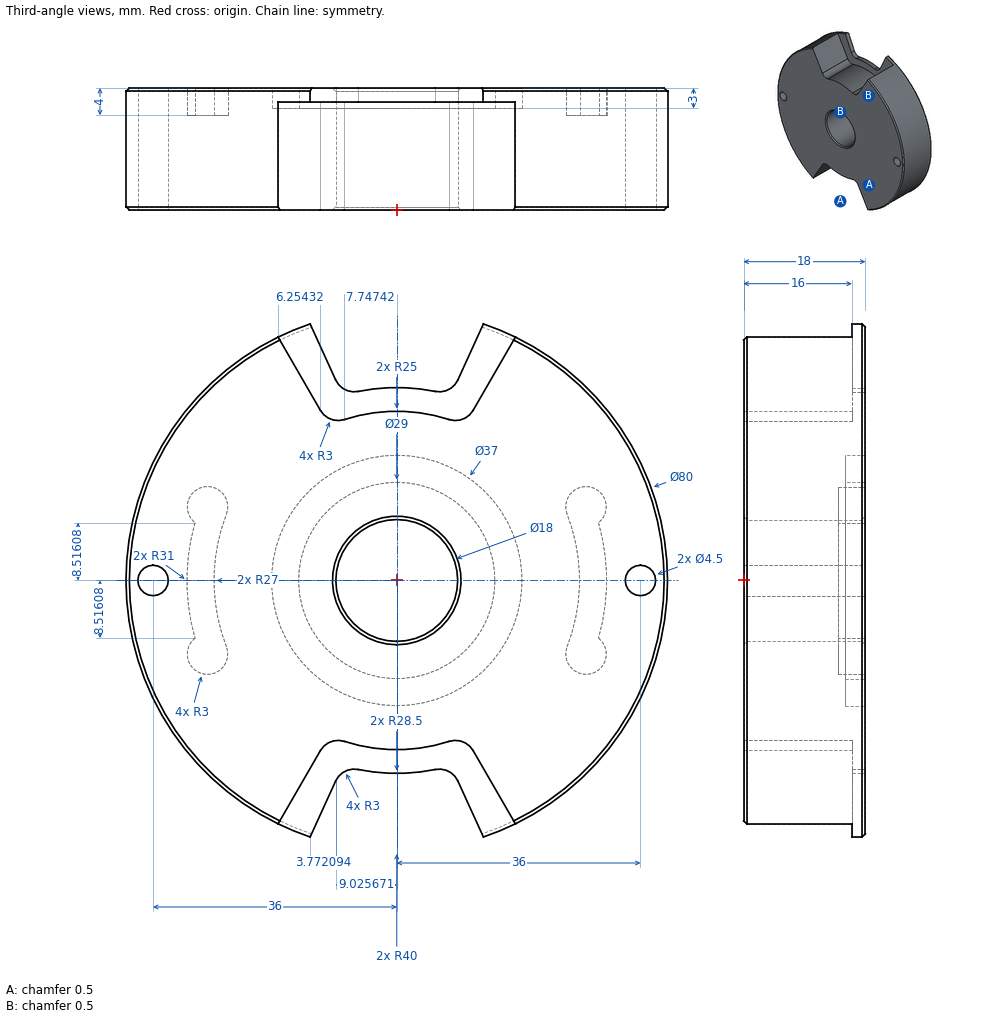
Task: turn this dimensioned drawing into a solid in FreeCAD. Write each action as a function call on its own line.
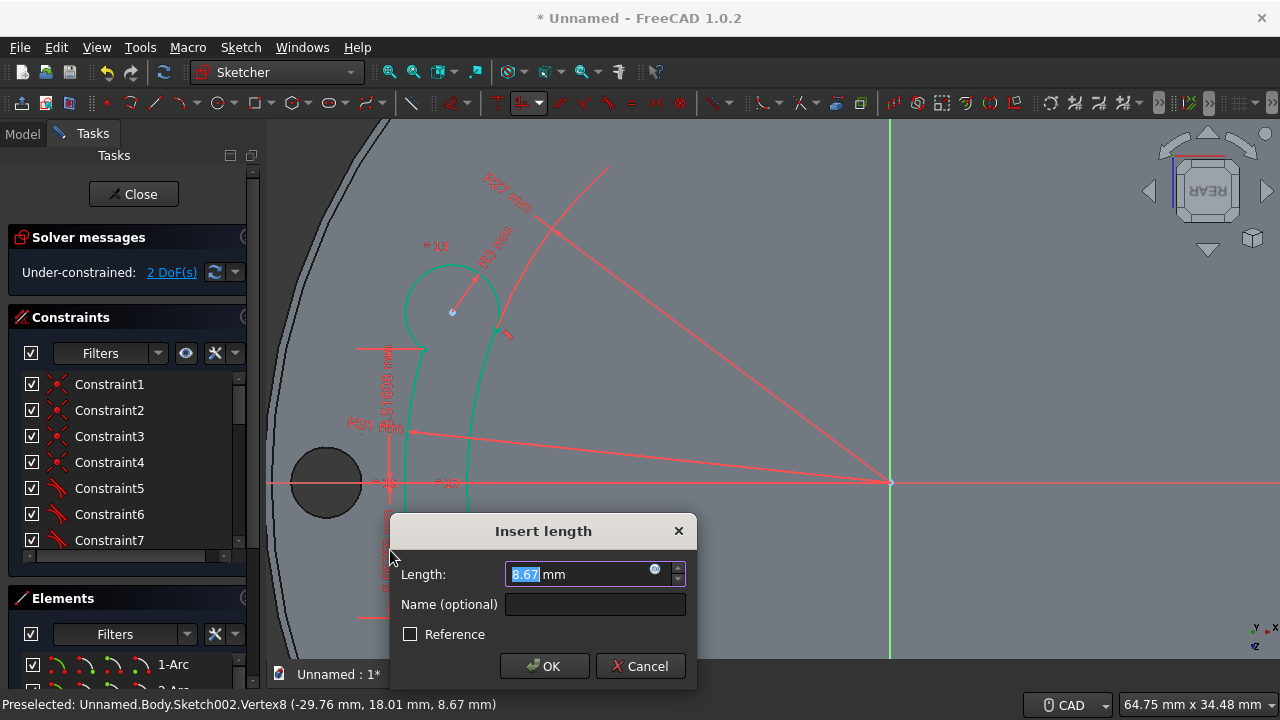
text(8.51608)
key(Return)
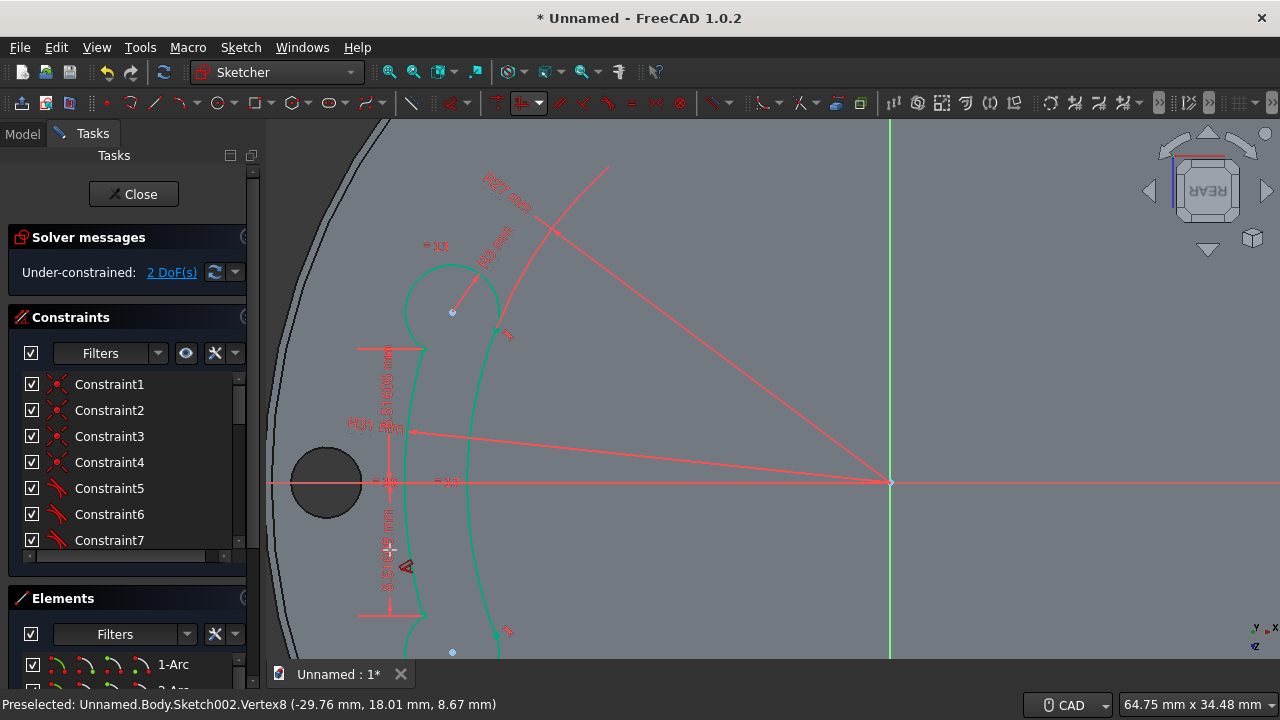
scroll(479, 275, down, 3)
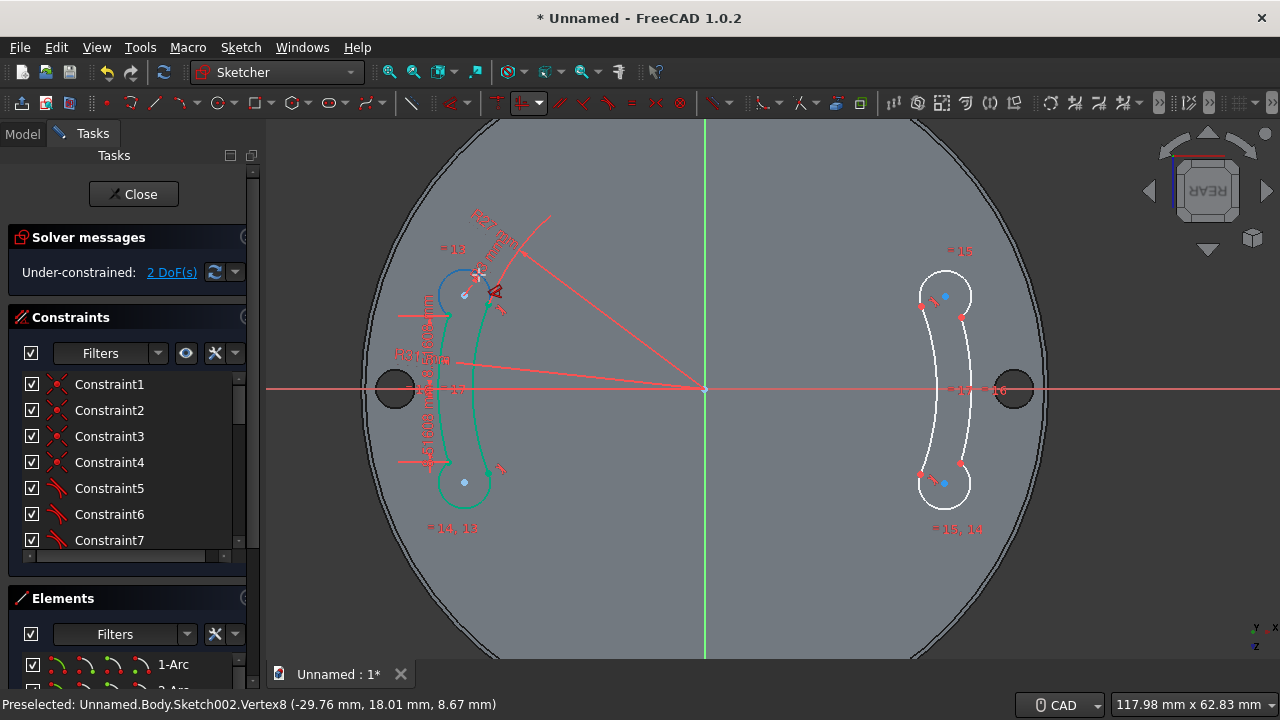
click(961, 463)
click(995, 426)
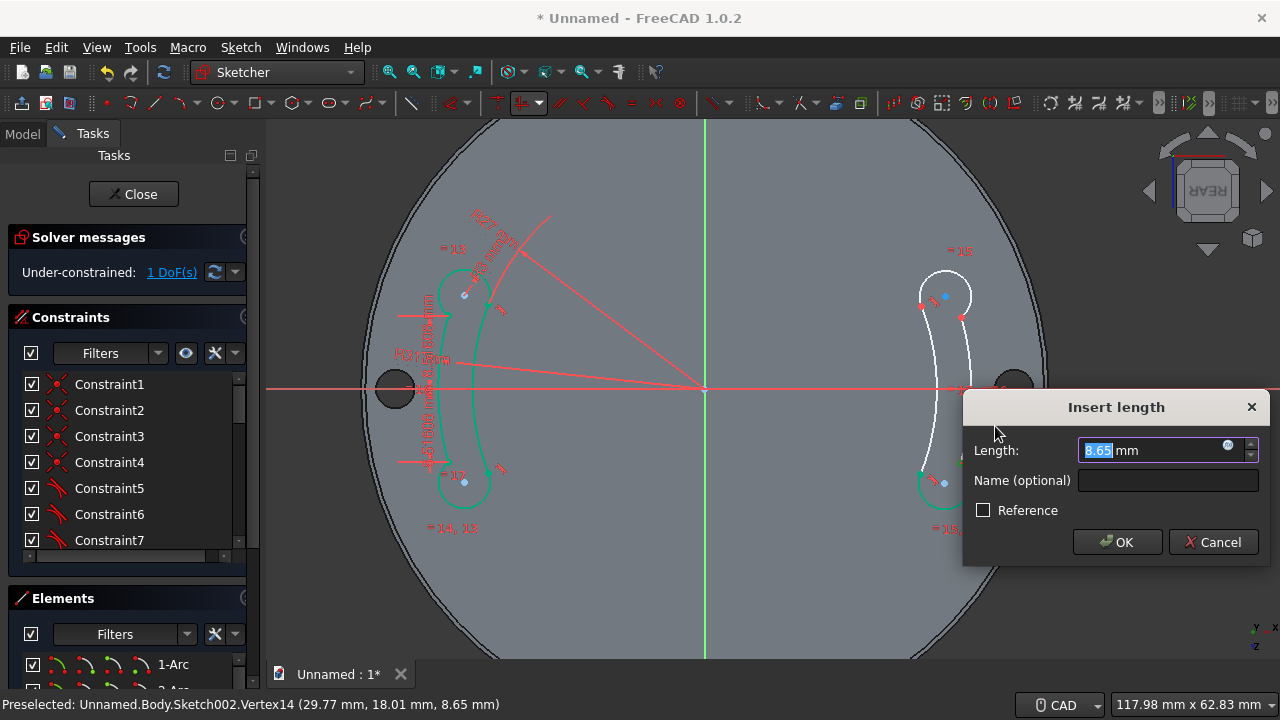
text(8.51608)
key(Return)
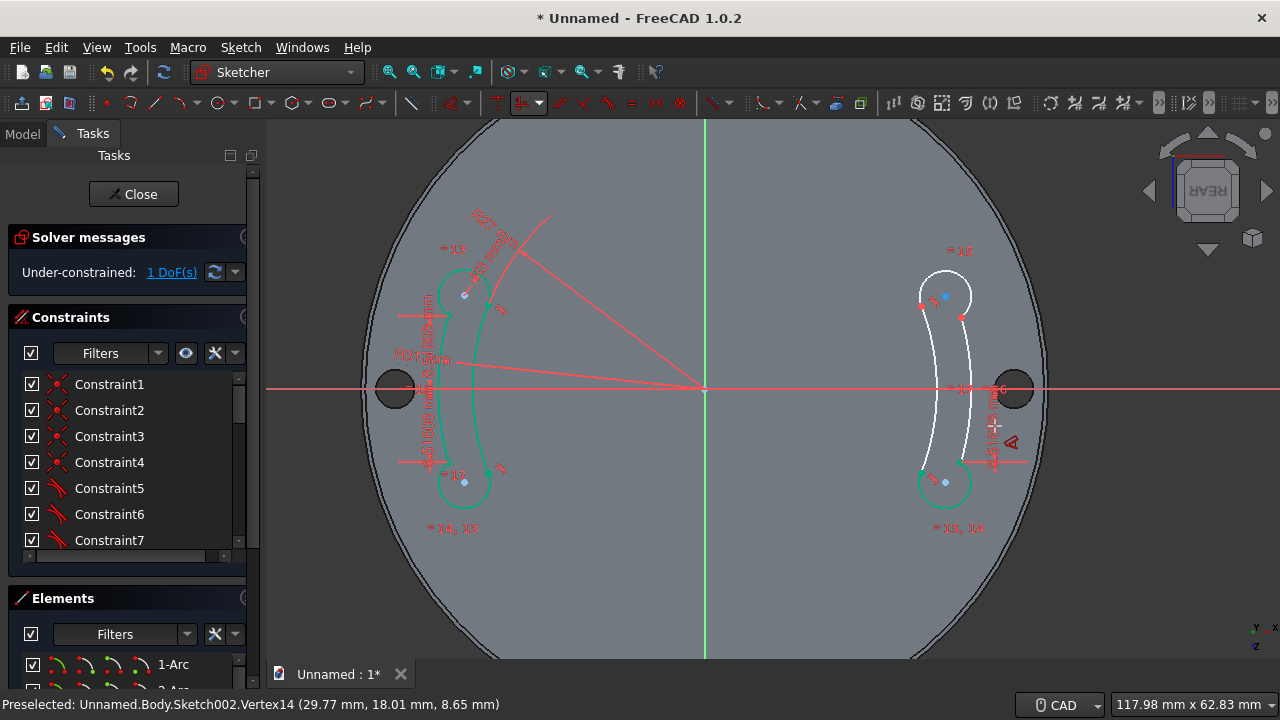
click(961, 317)
click(995, 353)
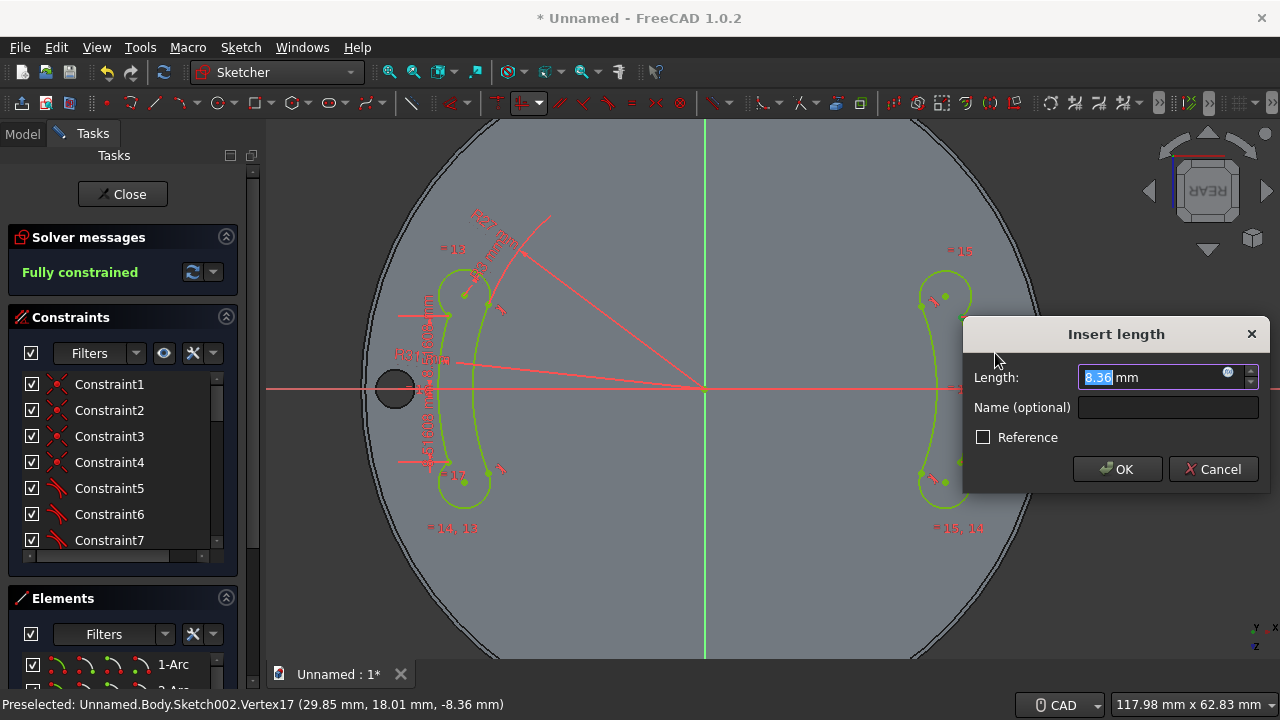
text(8.51608)
key(Return)
key(Escape)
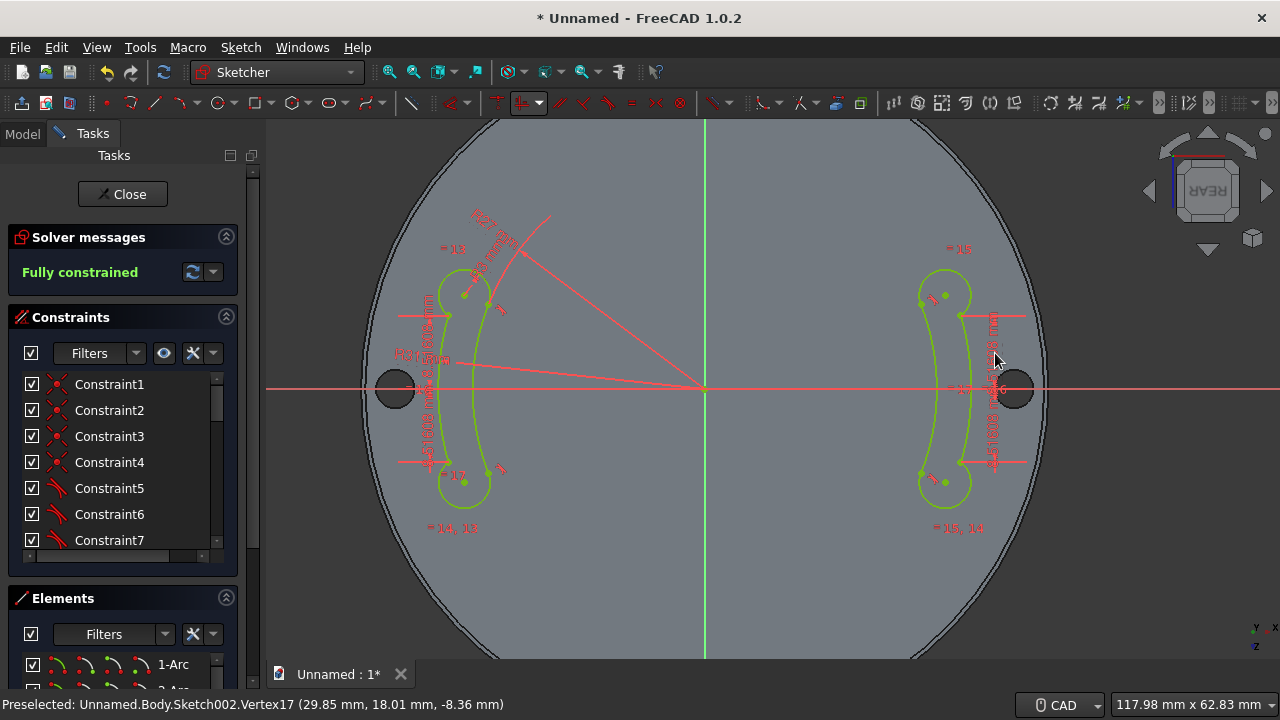
click(123, 194)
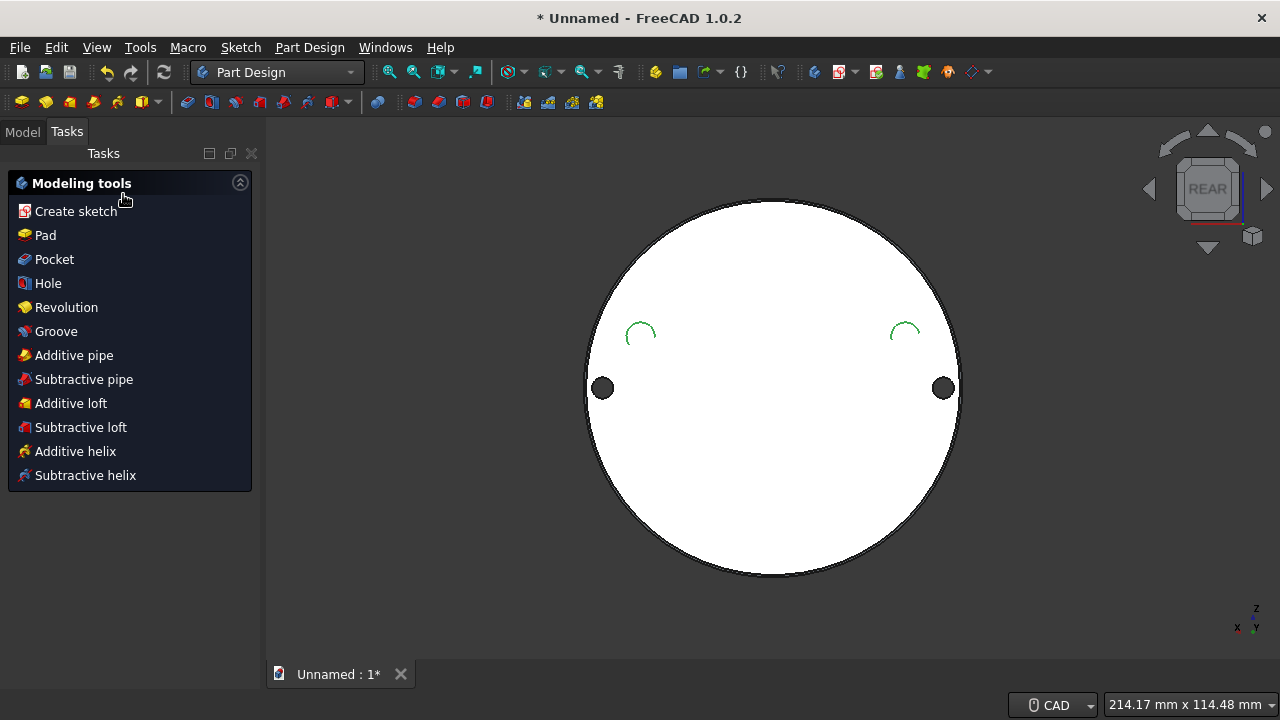
click(188, 102)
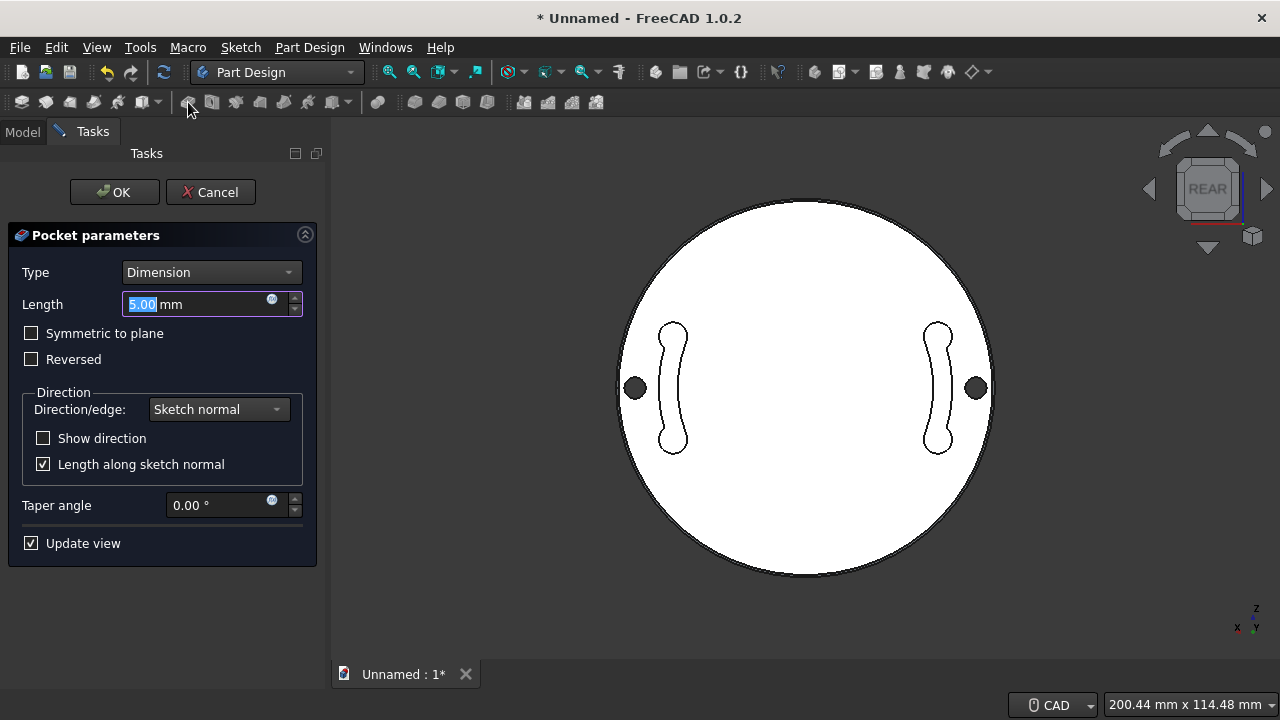
text(4)
key(Tab)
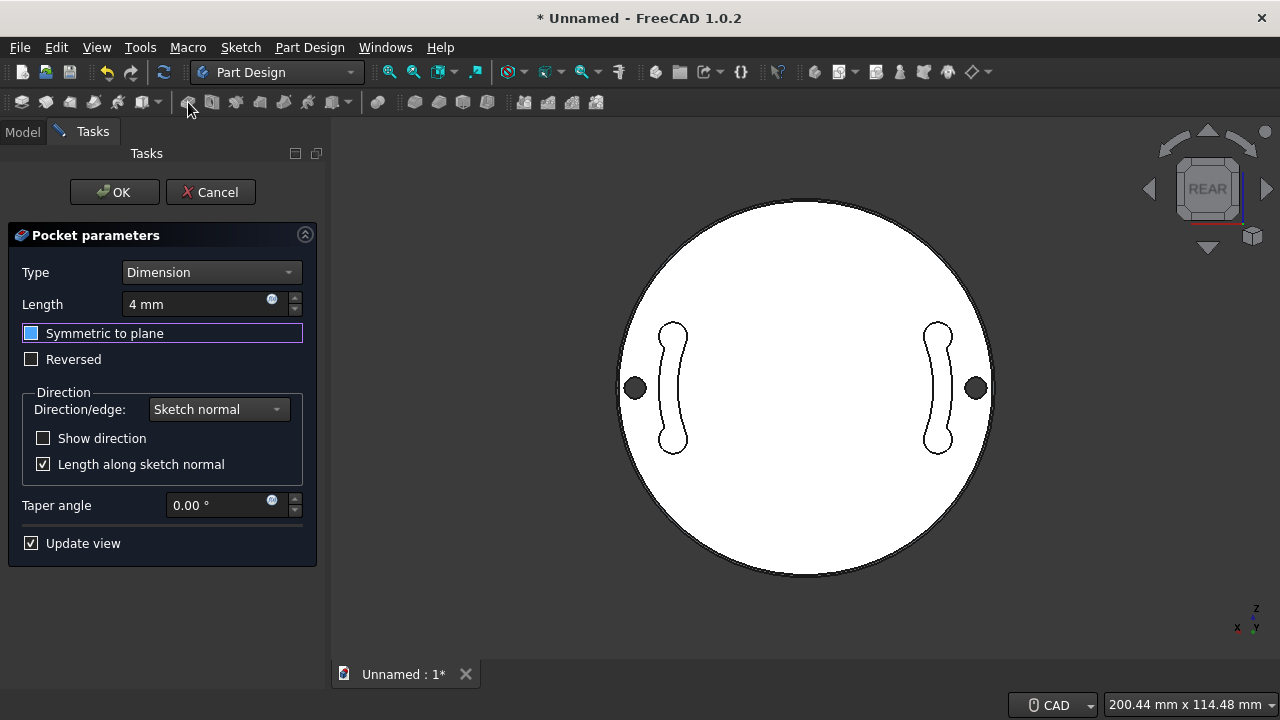
click(115, 192)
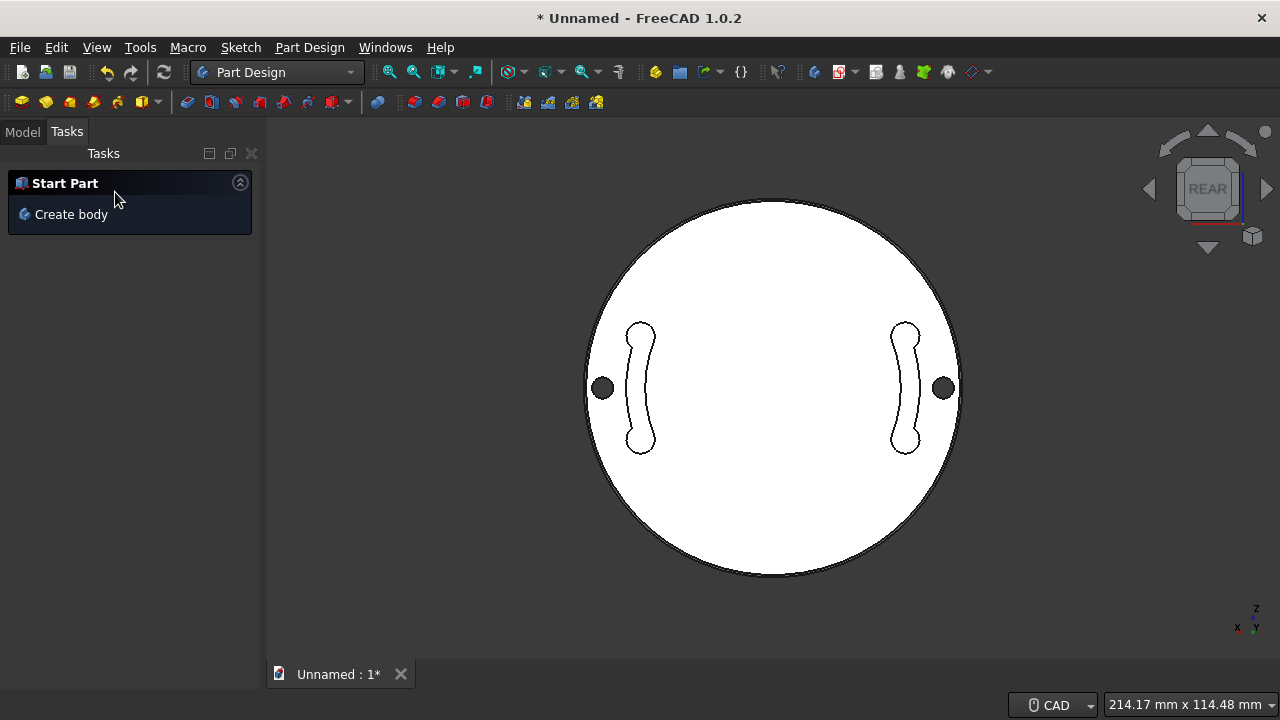
click(773, 387)